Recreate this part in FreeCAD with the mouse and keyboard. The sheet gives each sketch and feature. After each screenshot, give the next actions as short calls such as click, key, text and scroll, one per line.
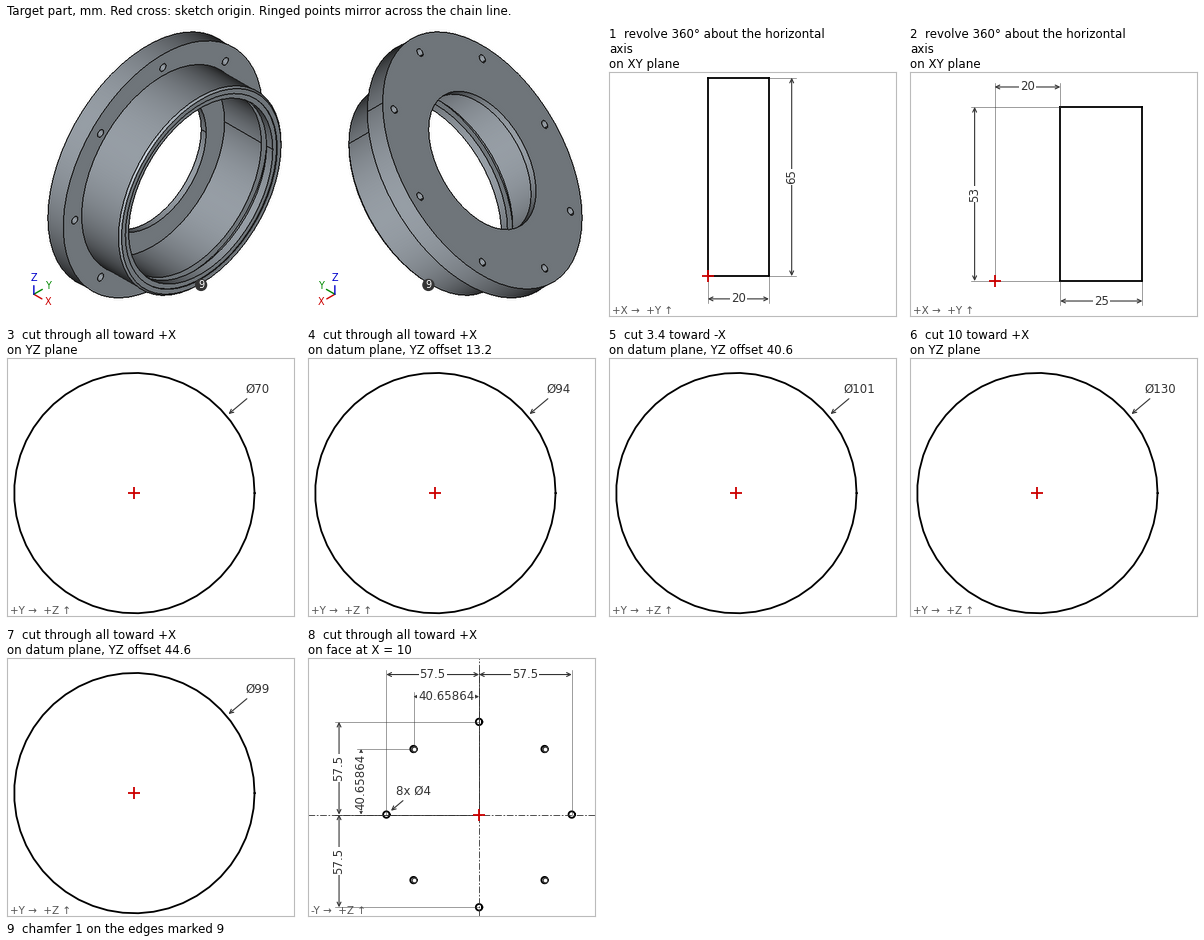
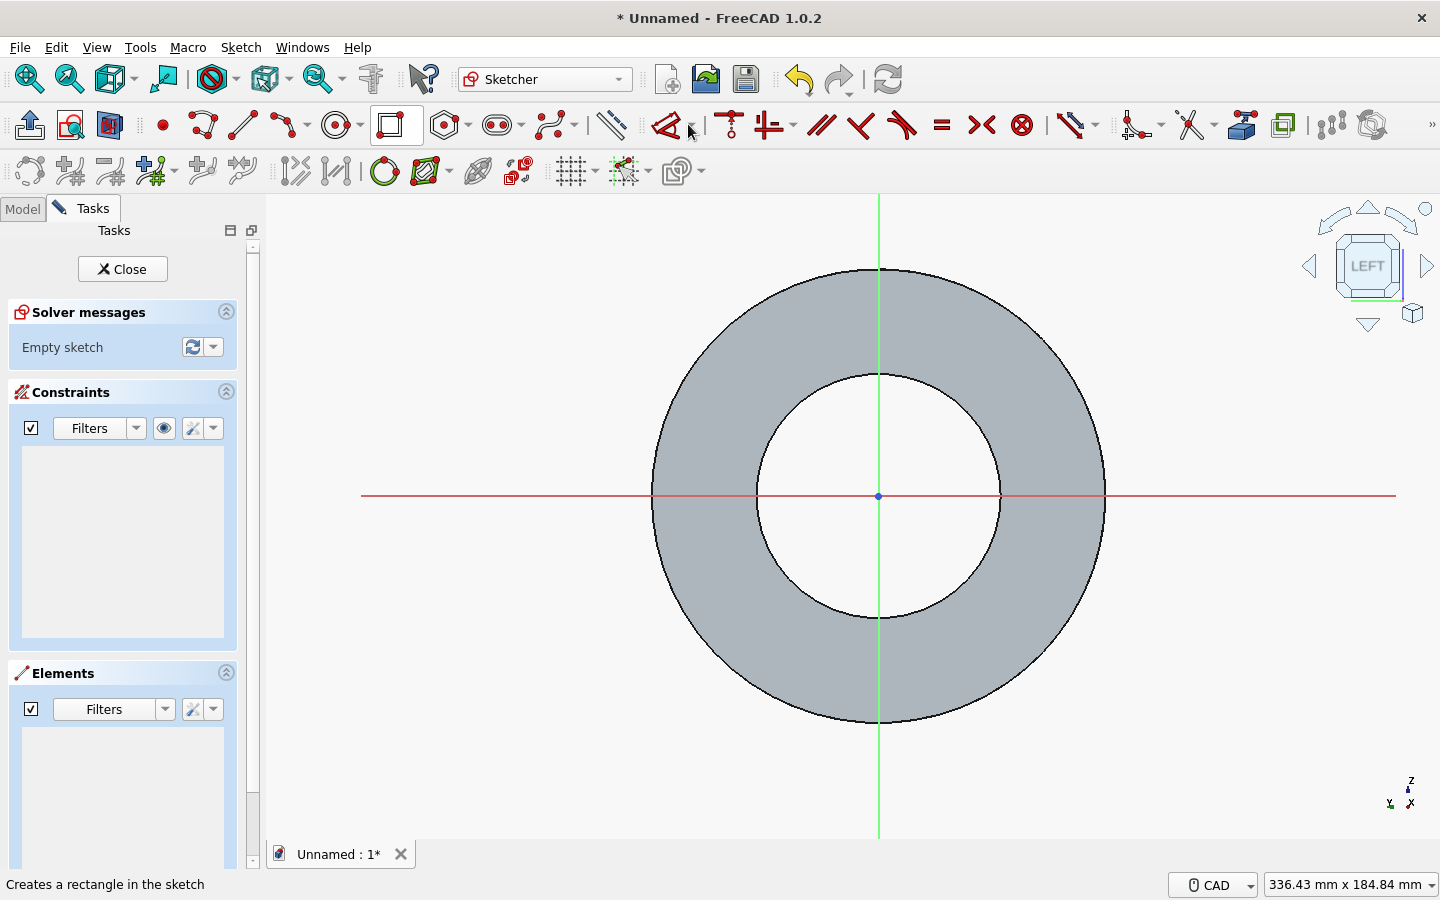
click(336, 126)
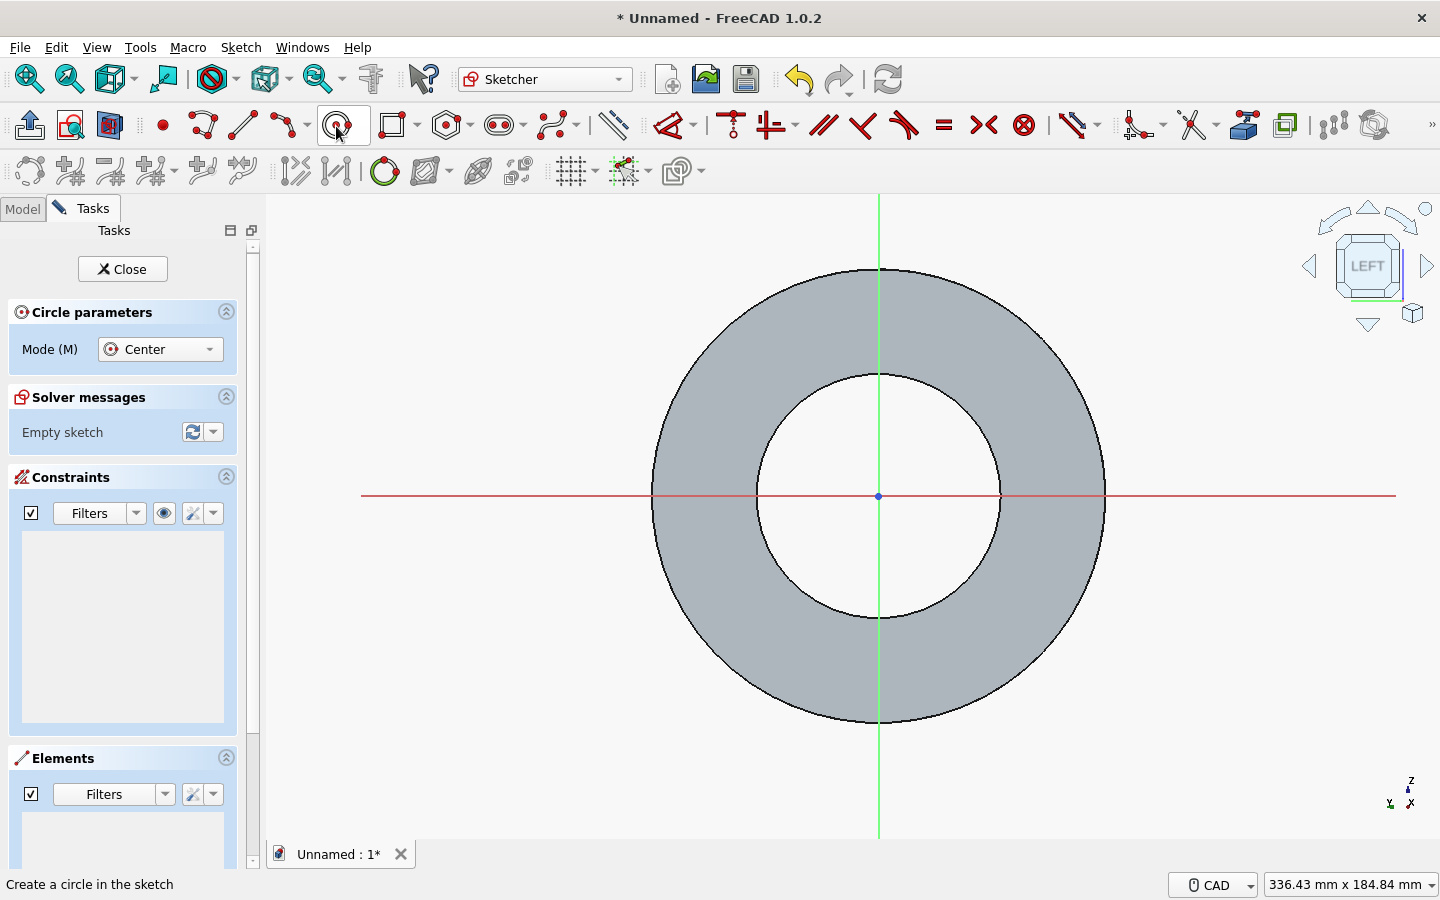
scroll(678, 496, up, 6)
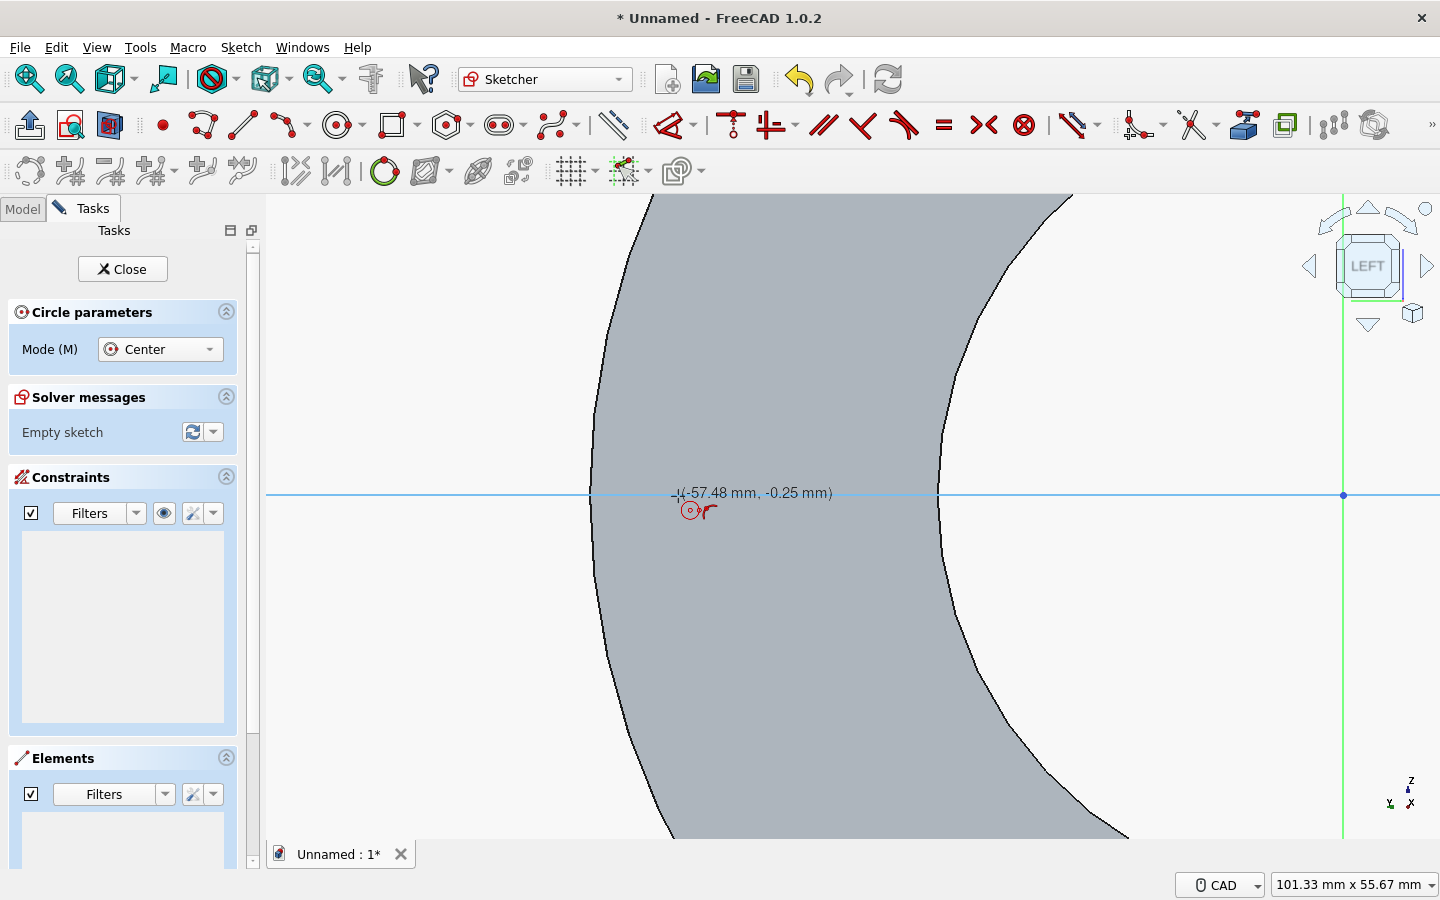
click(677, 495)
click(693, 479)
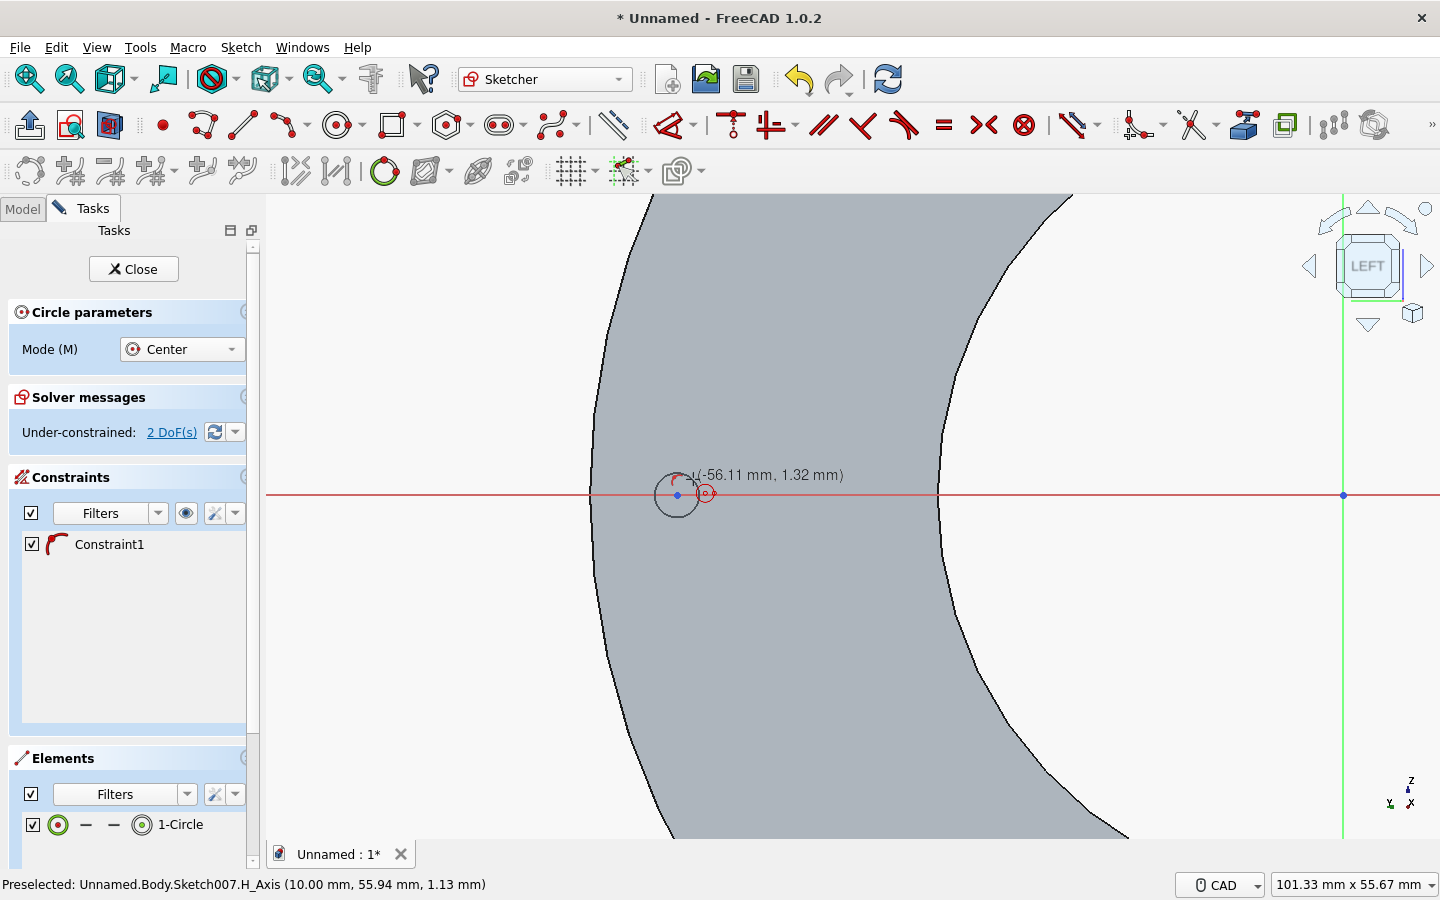
scroll(544, 526, down, 6)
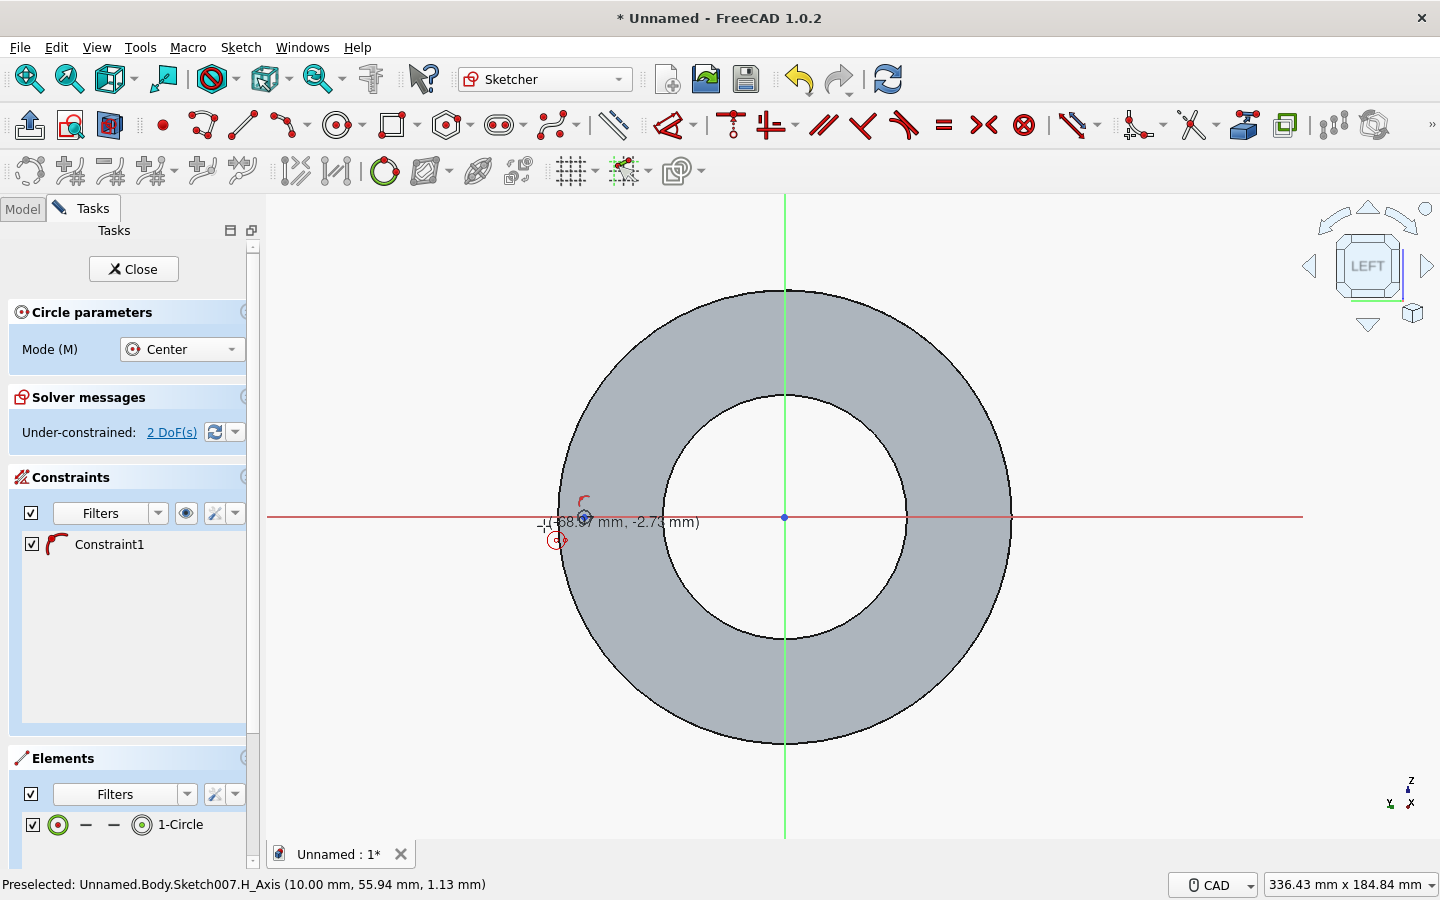
scroll(643, 375, up, 6)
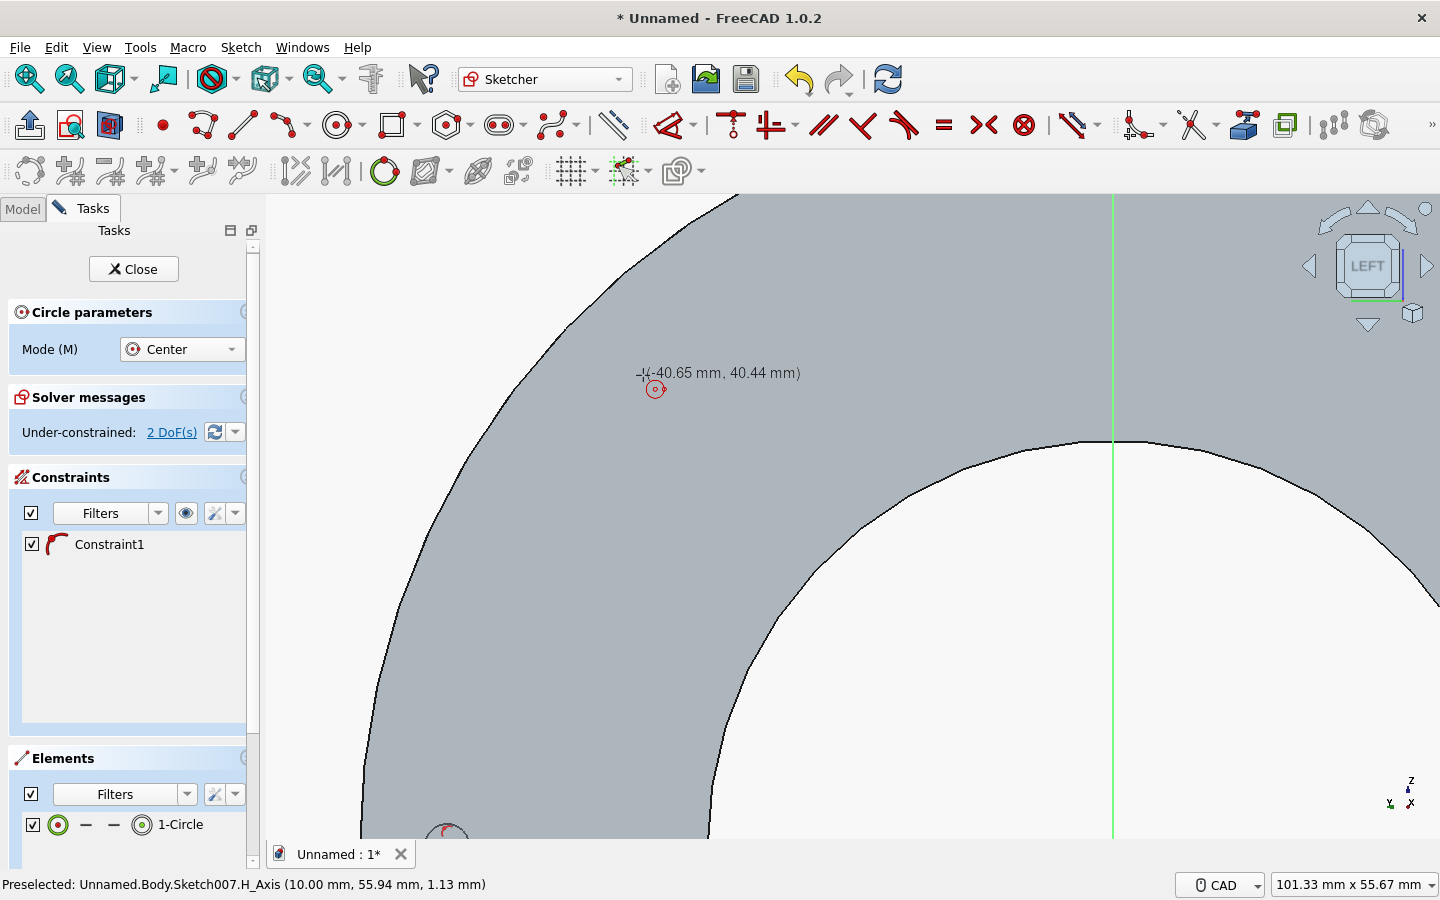
click(642, 375)
click(659, 359)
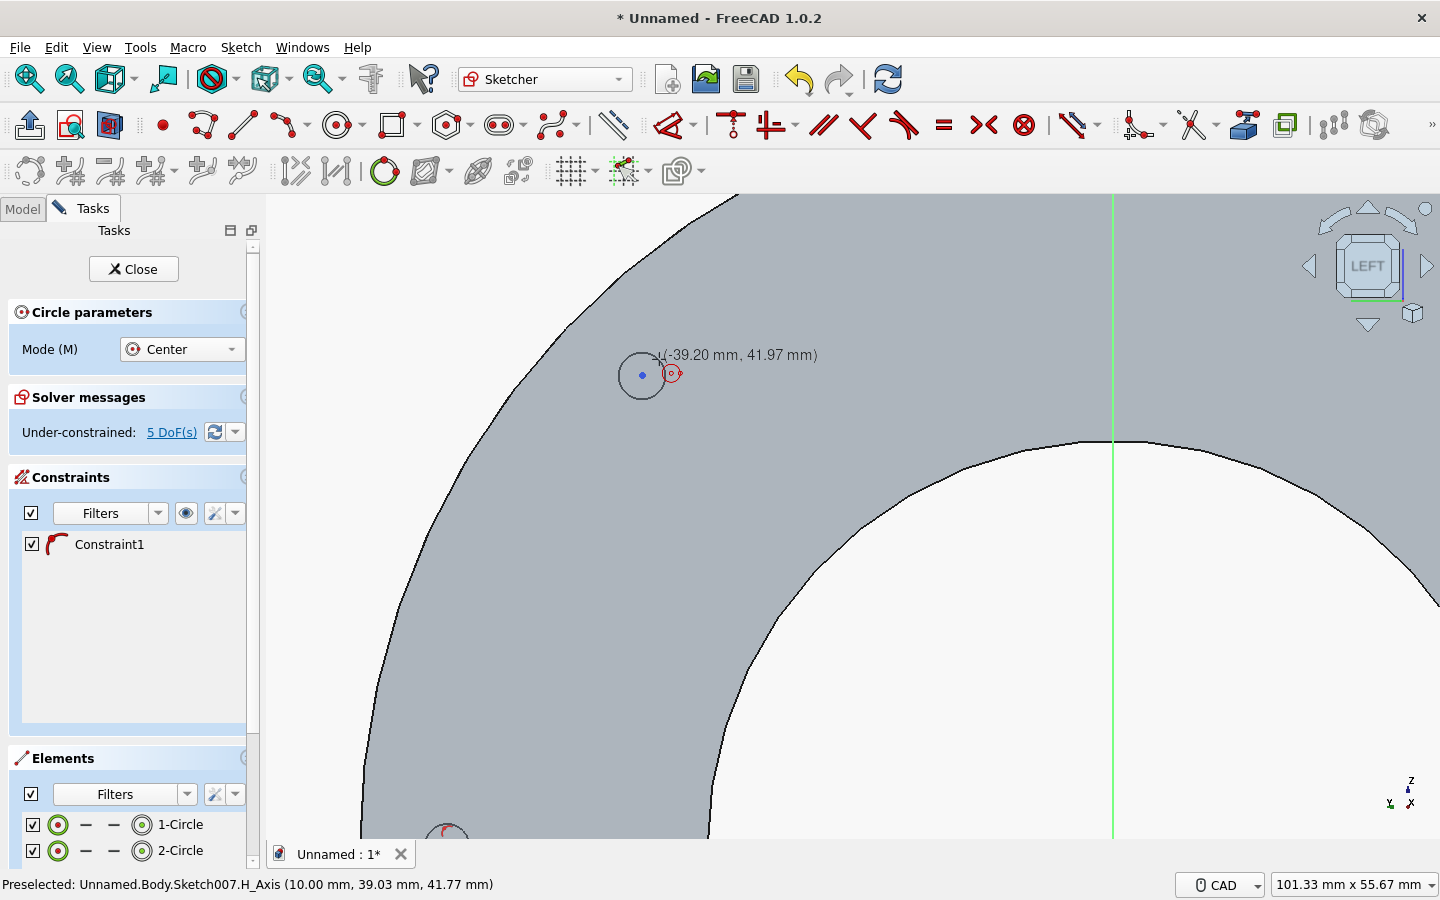
scroll(643, 374, down, 6)